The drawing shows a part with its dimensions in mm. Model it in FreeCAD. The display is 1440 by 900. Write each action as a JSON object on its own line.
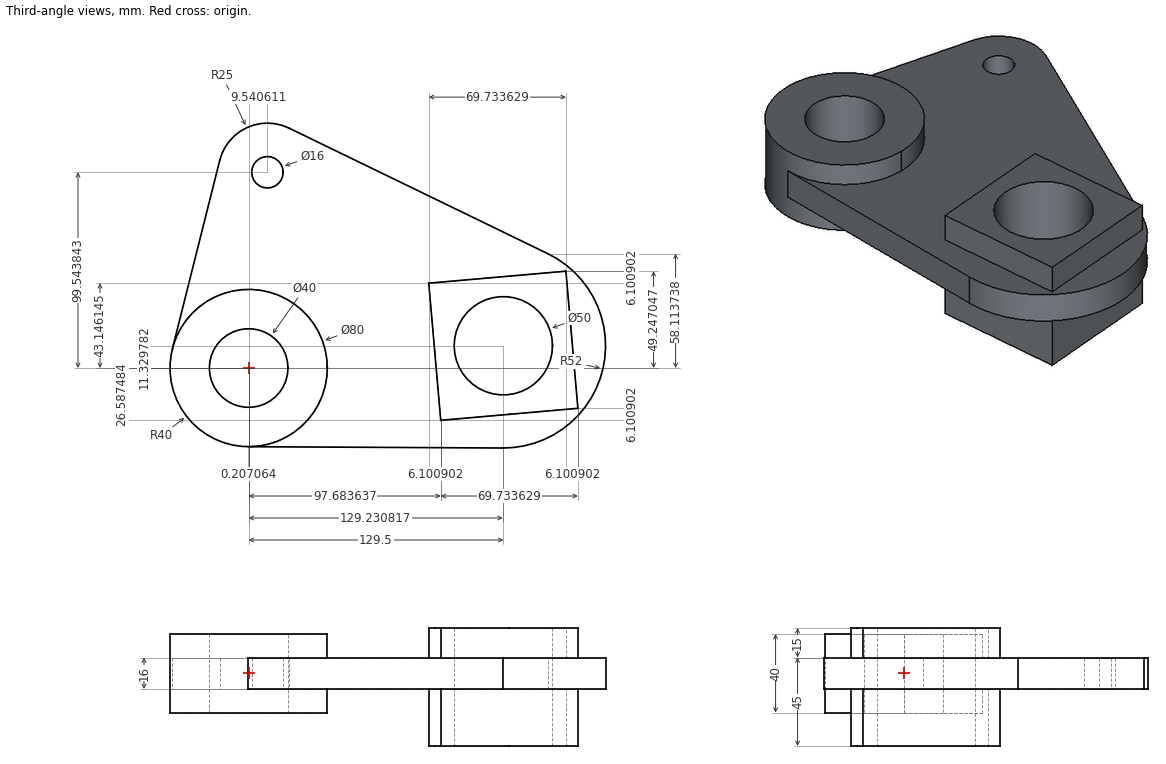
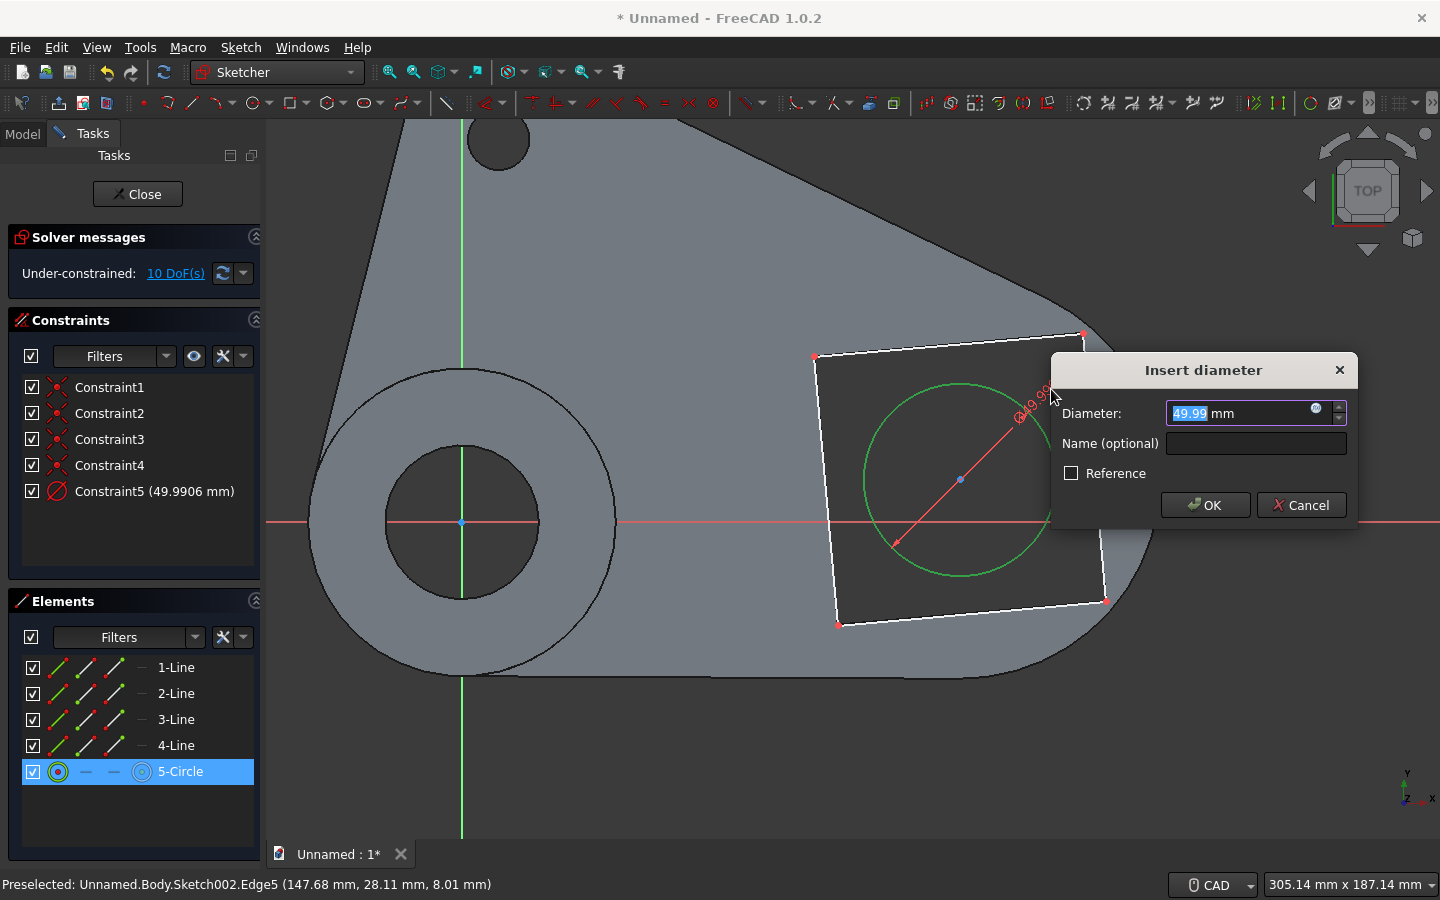
{"action": "type", "text": "50"}
{"action": "key", "text": "Return"}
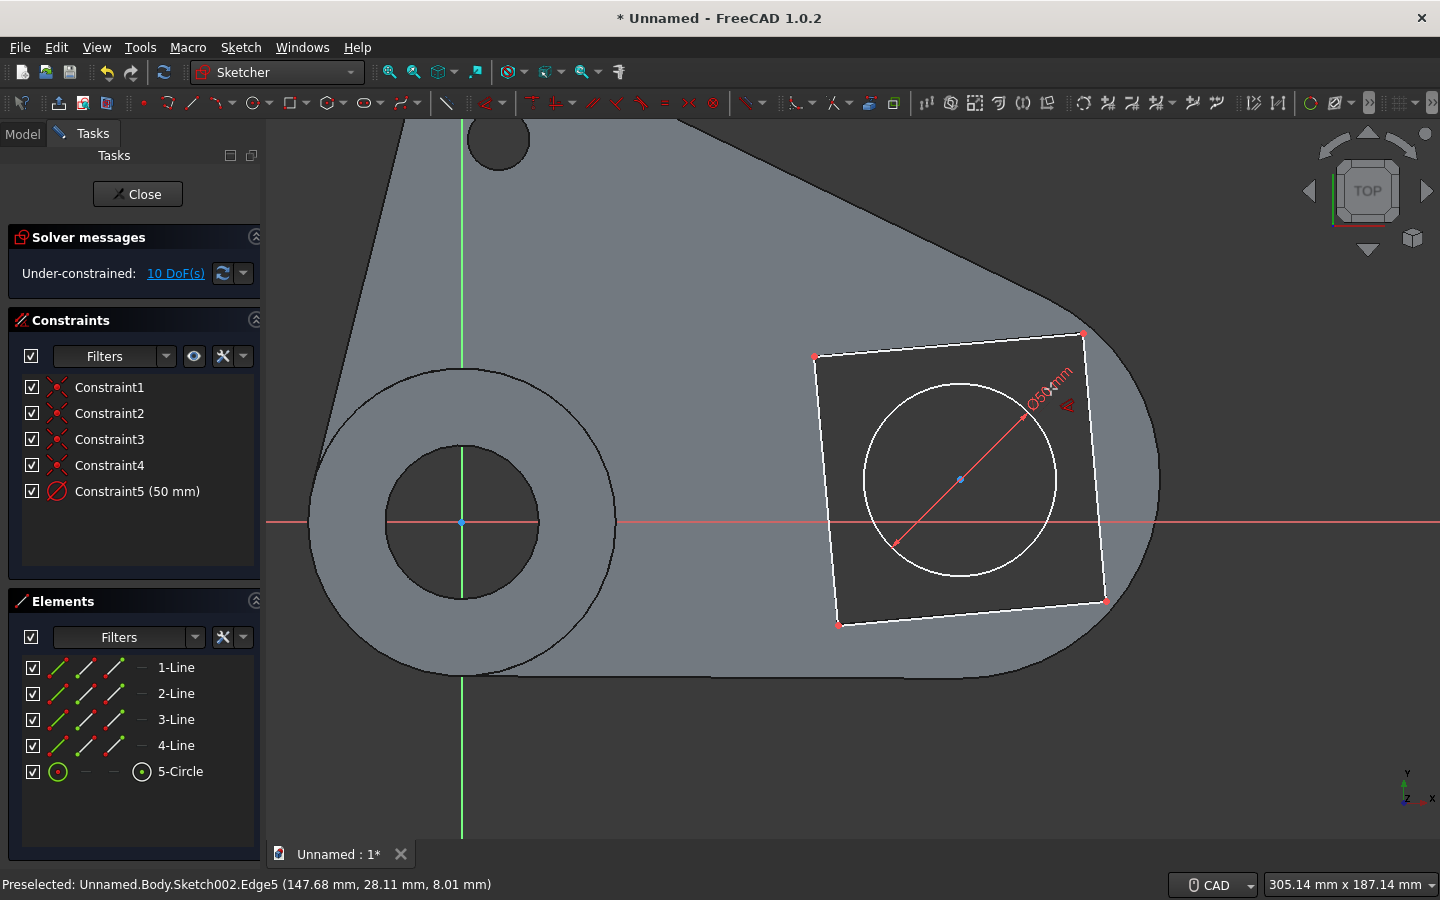
{"action": "left_click", "coordinate": [960, 480]}
{"action": "left_click", "coordinate": [711, 556]}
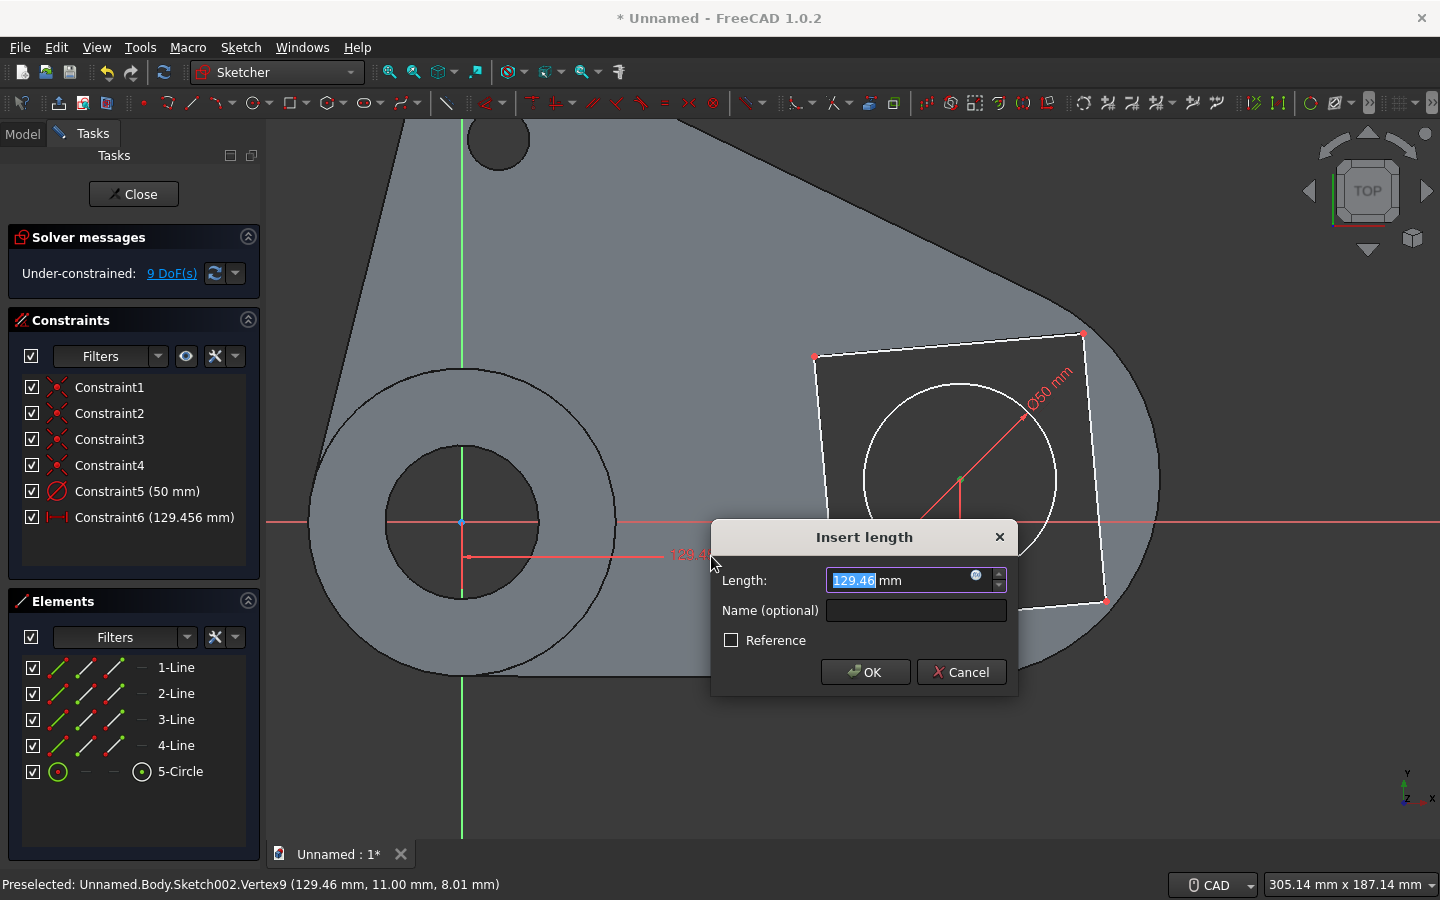
{"action": "type", "text": "129.5"}
{"action": "key", "text": "Return"}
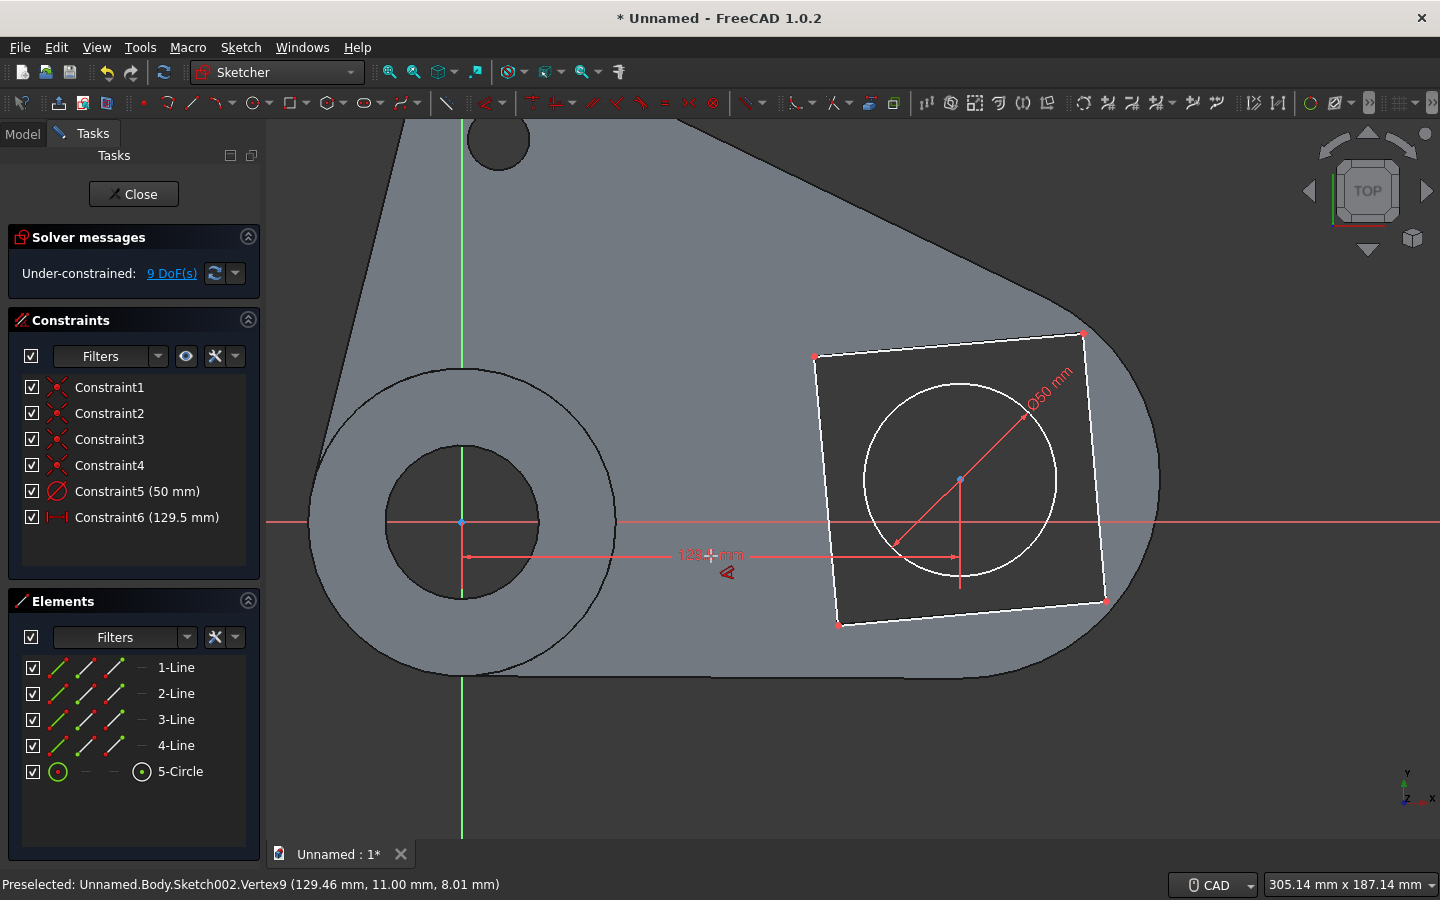
{"action": "scroll", "coordinate": [918, 619], "scroll_direction": "up", "scroll_amount": 3}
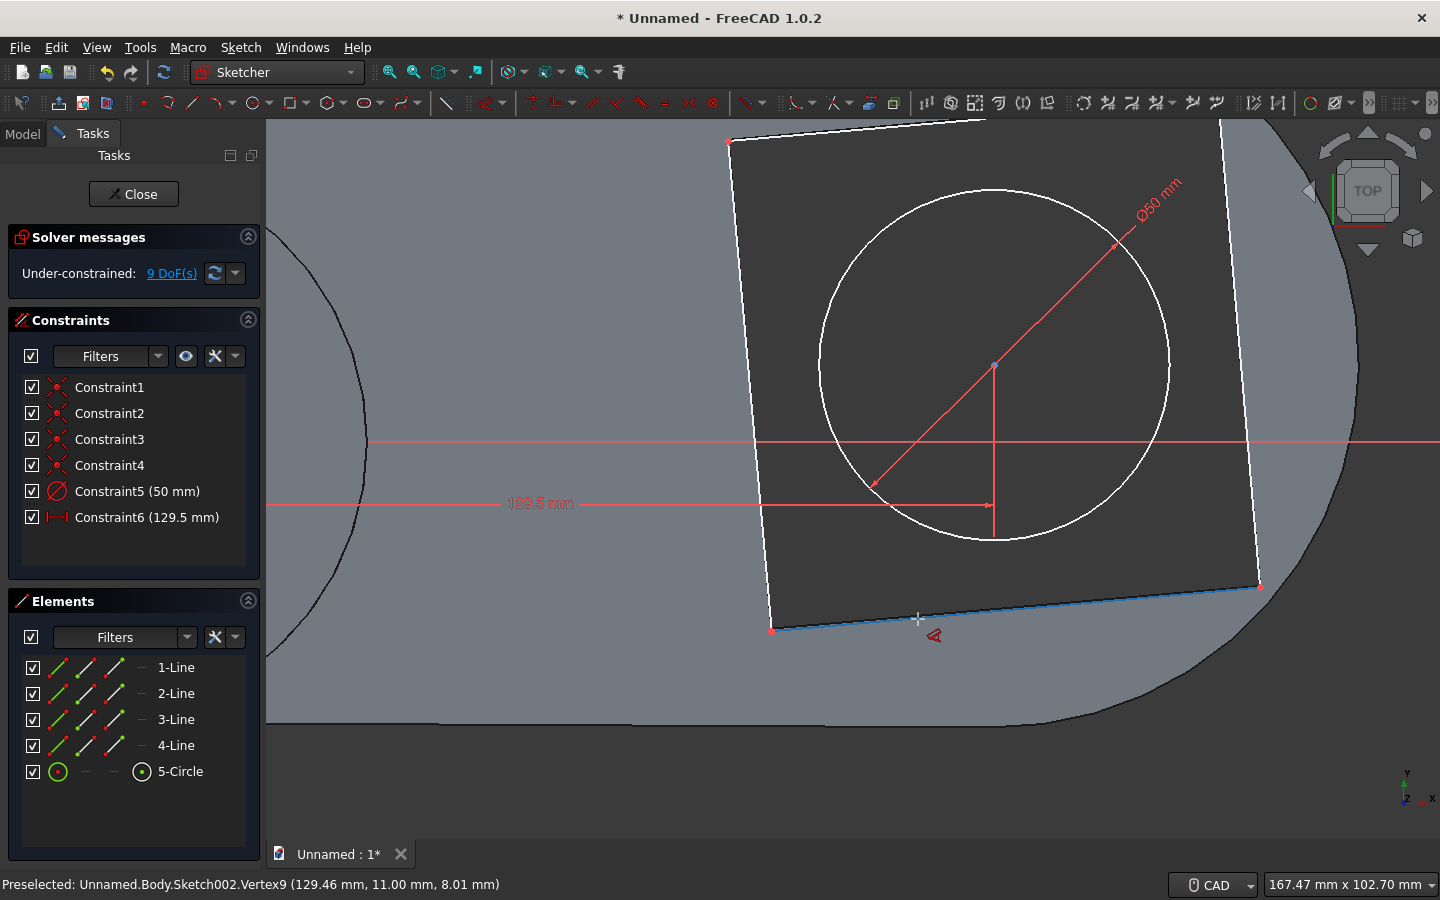
{"action": "left_click", "coordinate": [918, 618]}
{"action": "left_click", "coordinate": [738, 609]}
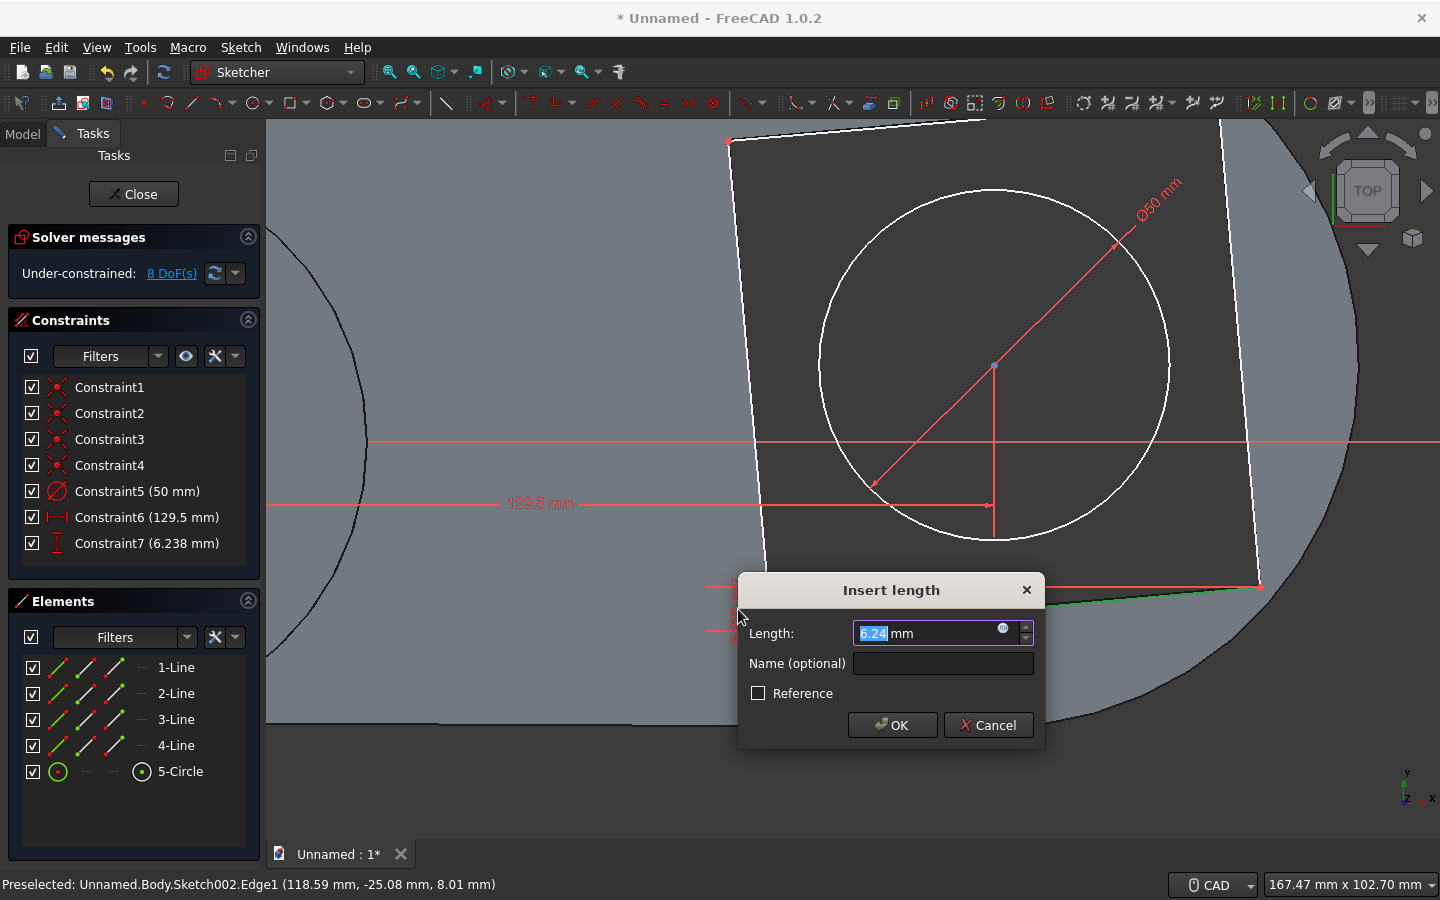
{"action": "type", "text": "6.100902"}
{"action": "key", "text": "Return"}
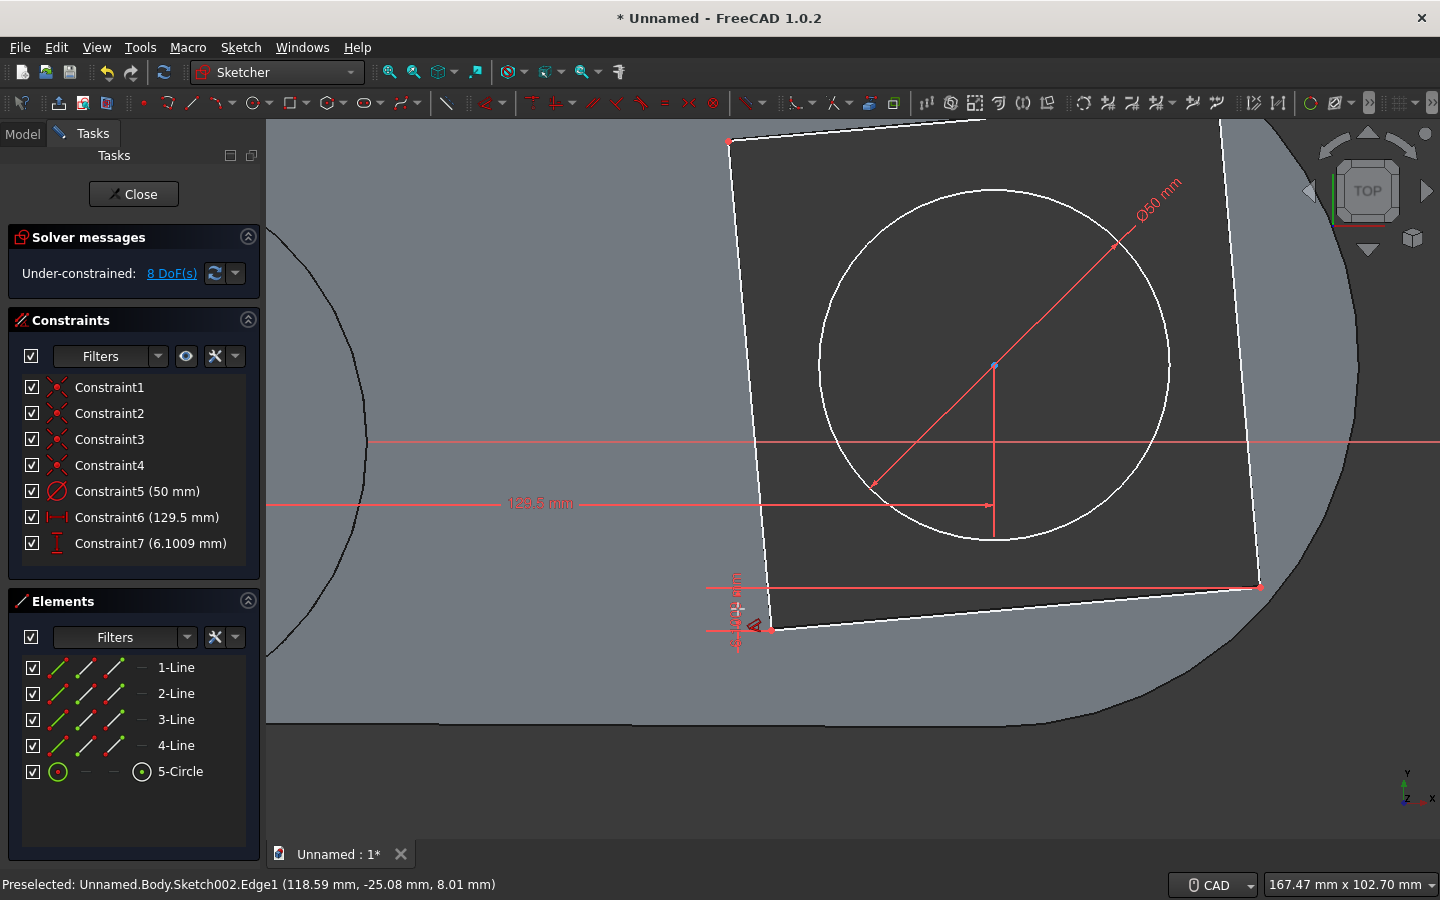
{"action": "left_click", "coordinate": [1248, 441]}
{"action": "left_click", "coordinate": [1239, 622]}